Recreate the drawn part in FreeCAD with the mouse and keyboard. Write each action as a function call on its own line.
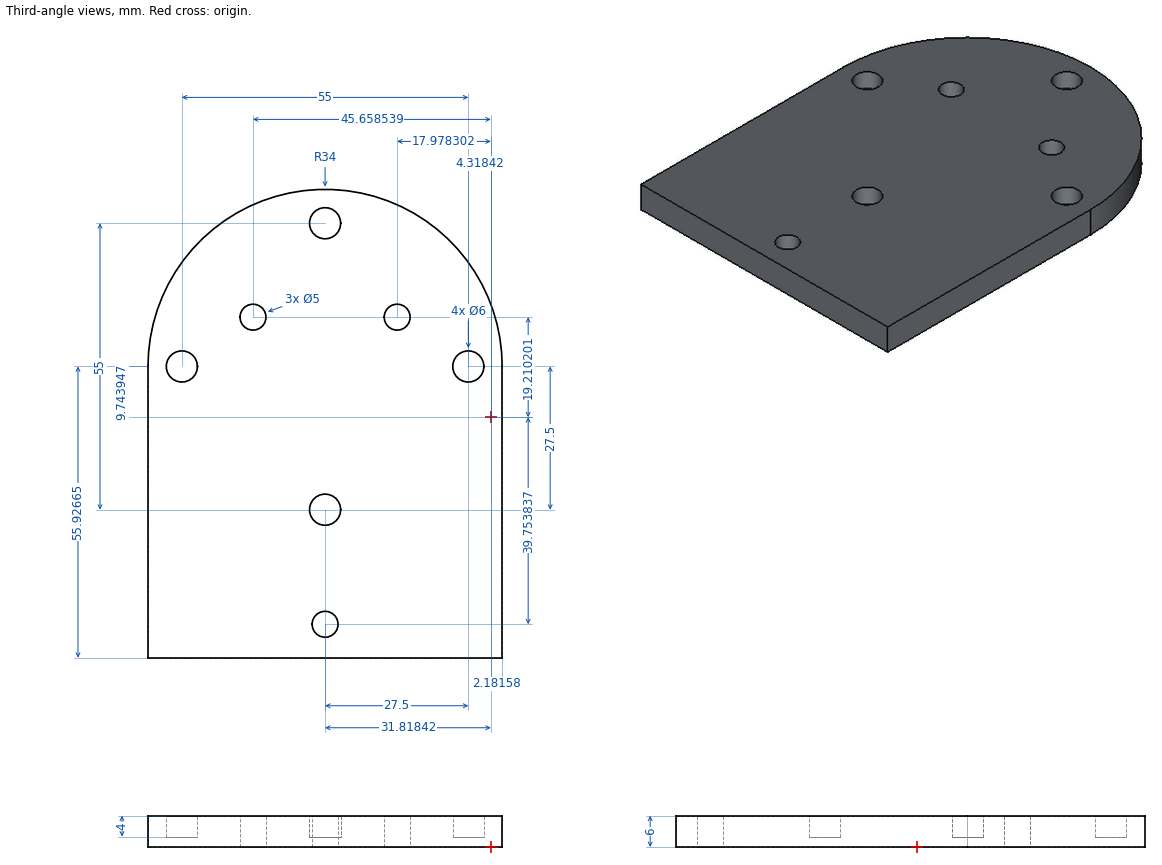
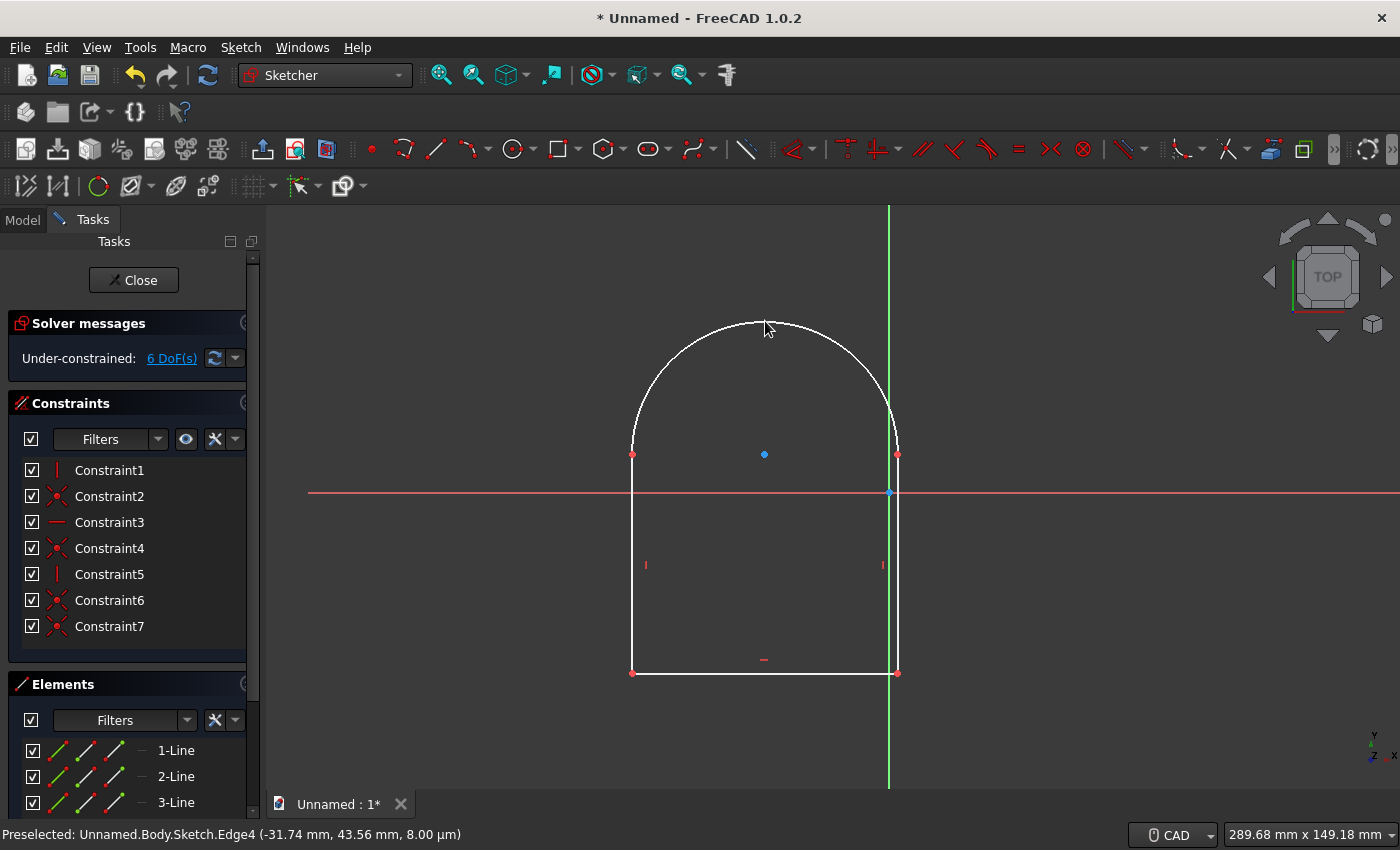
click(632, 521)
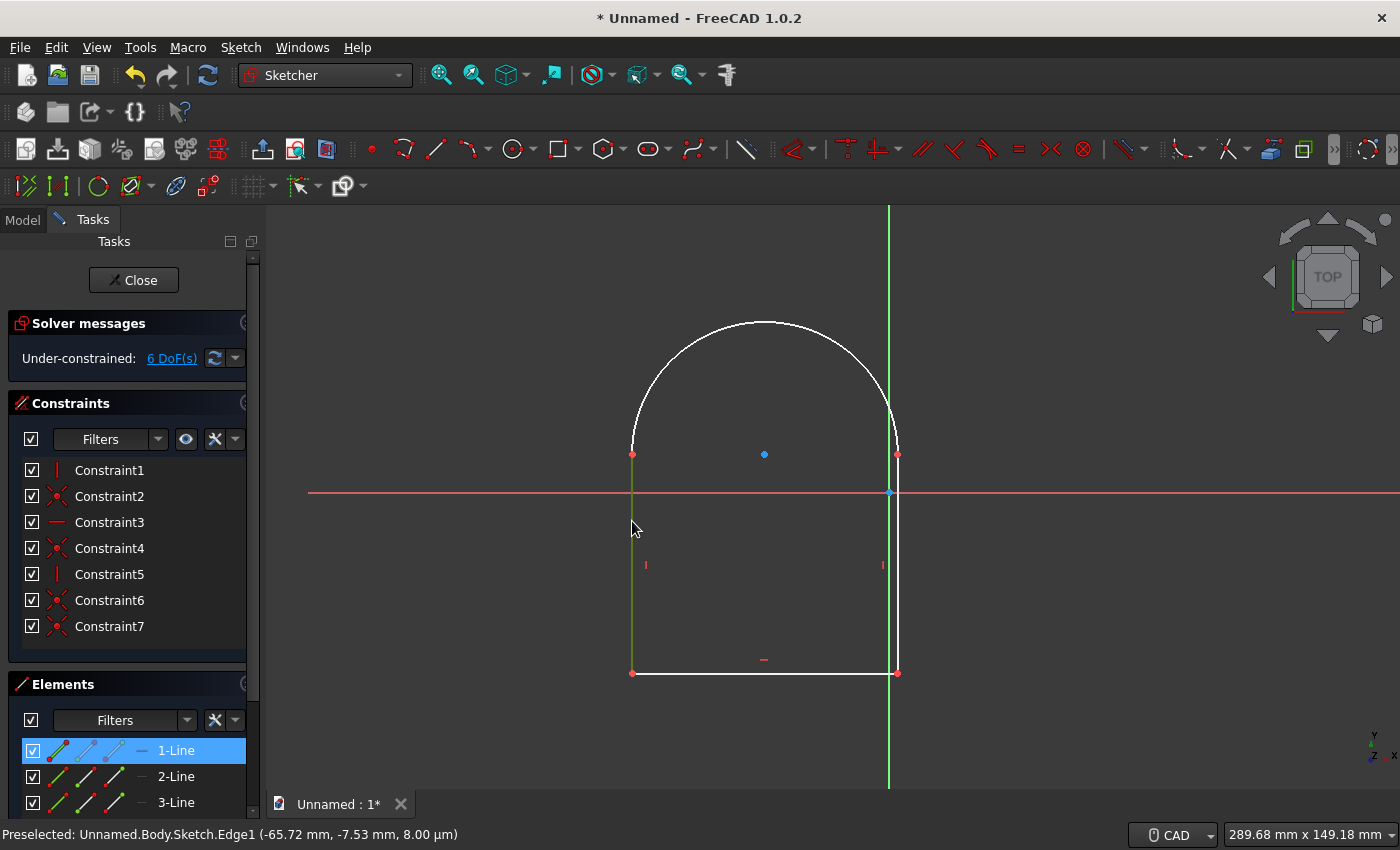
click(843, 347)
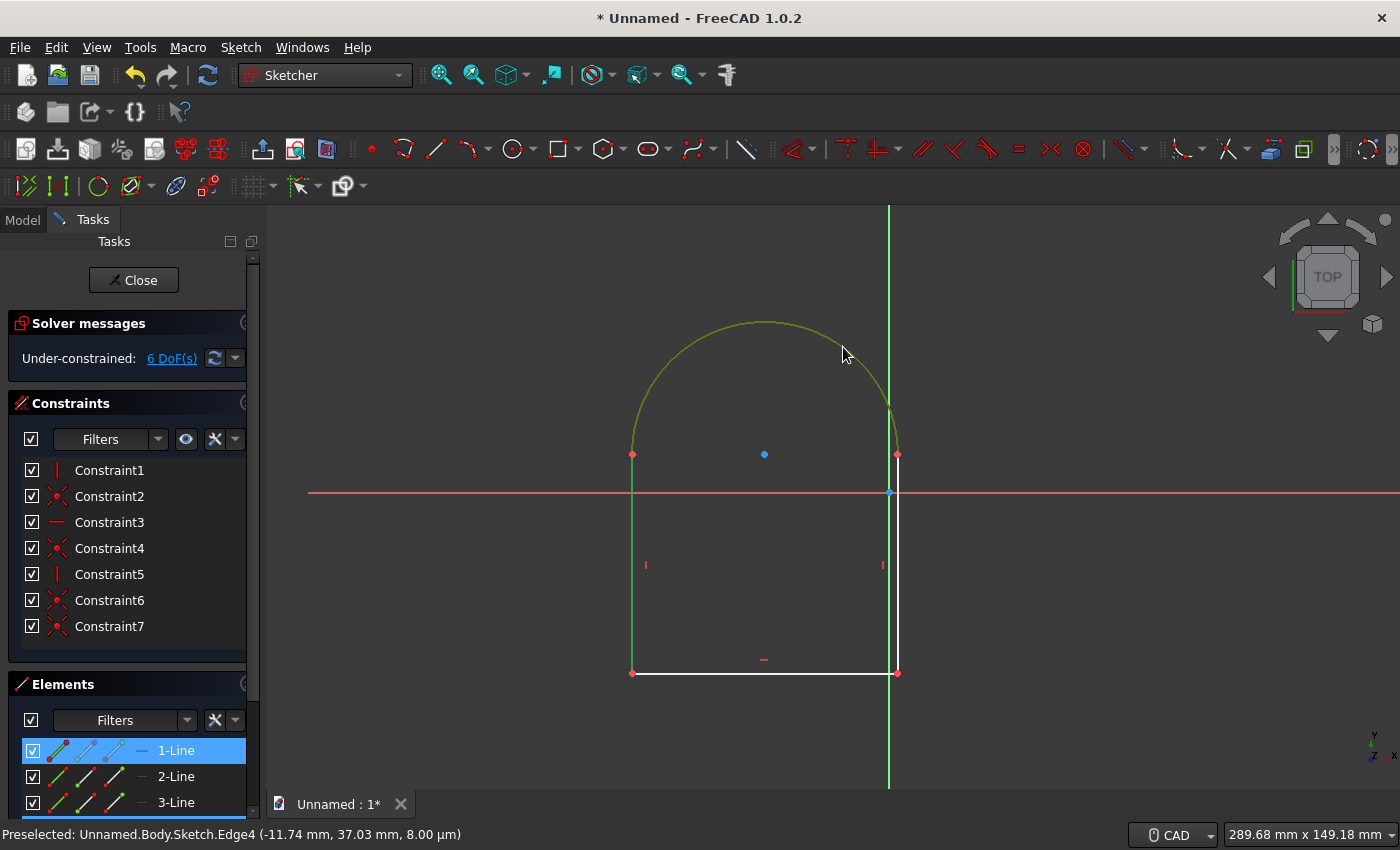
key(t)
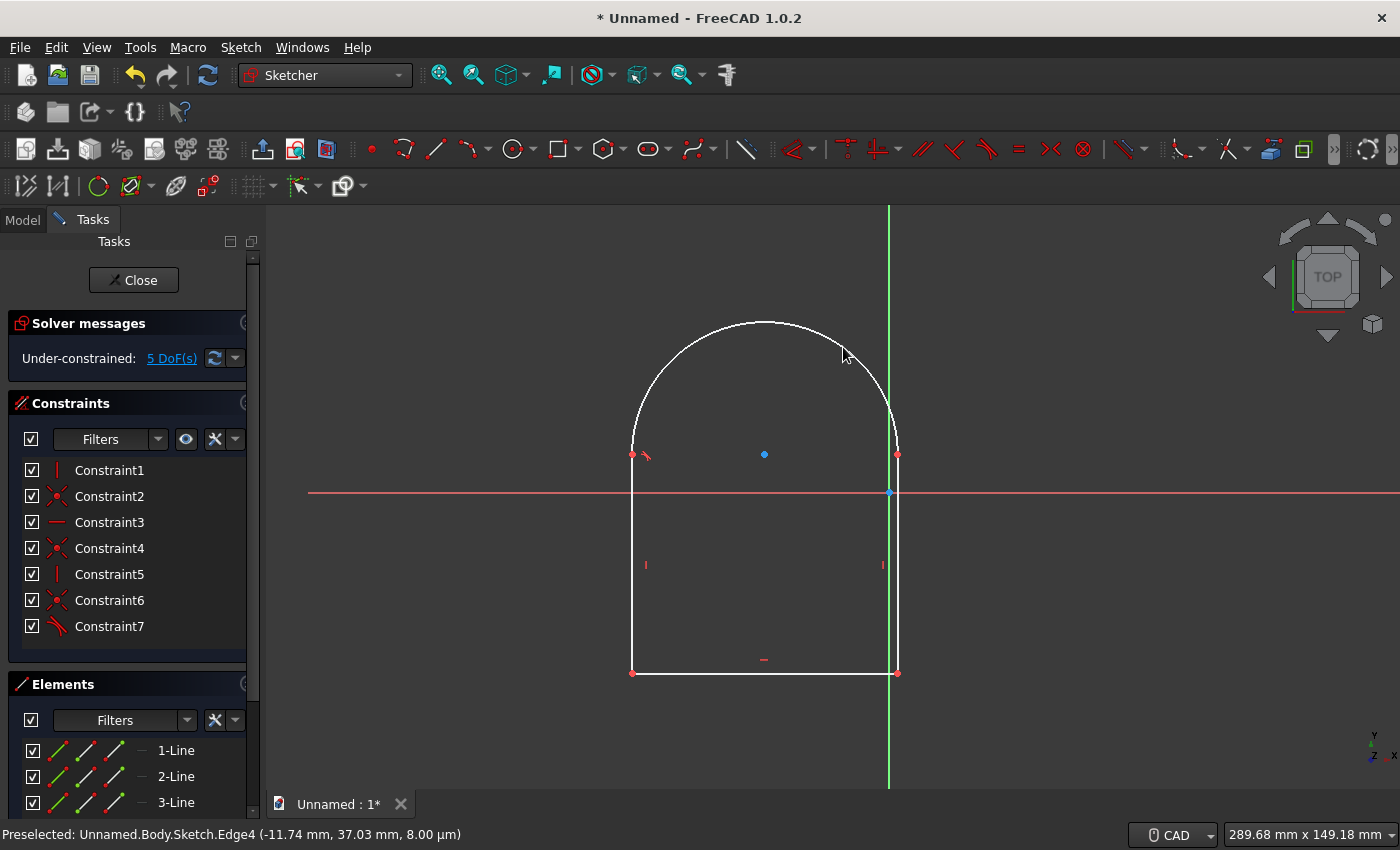
scroll(898, 608, up, 3)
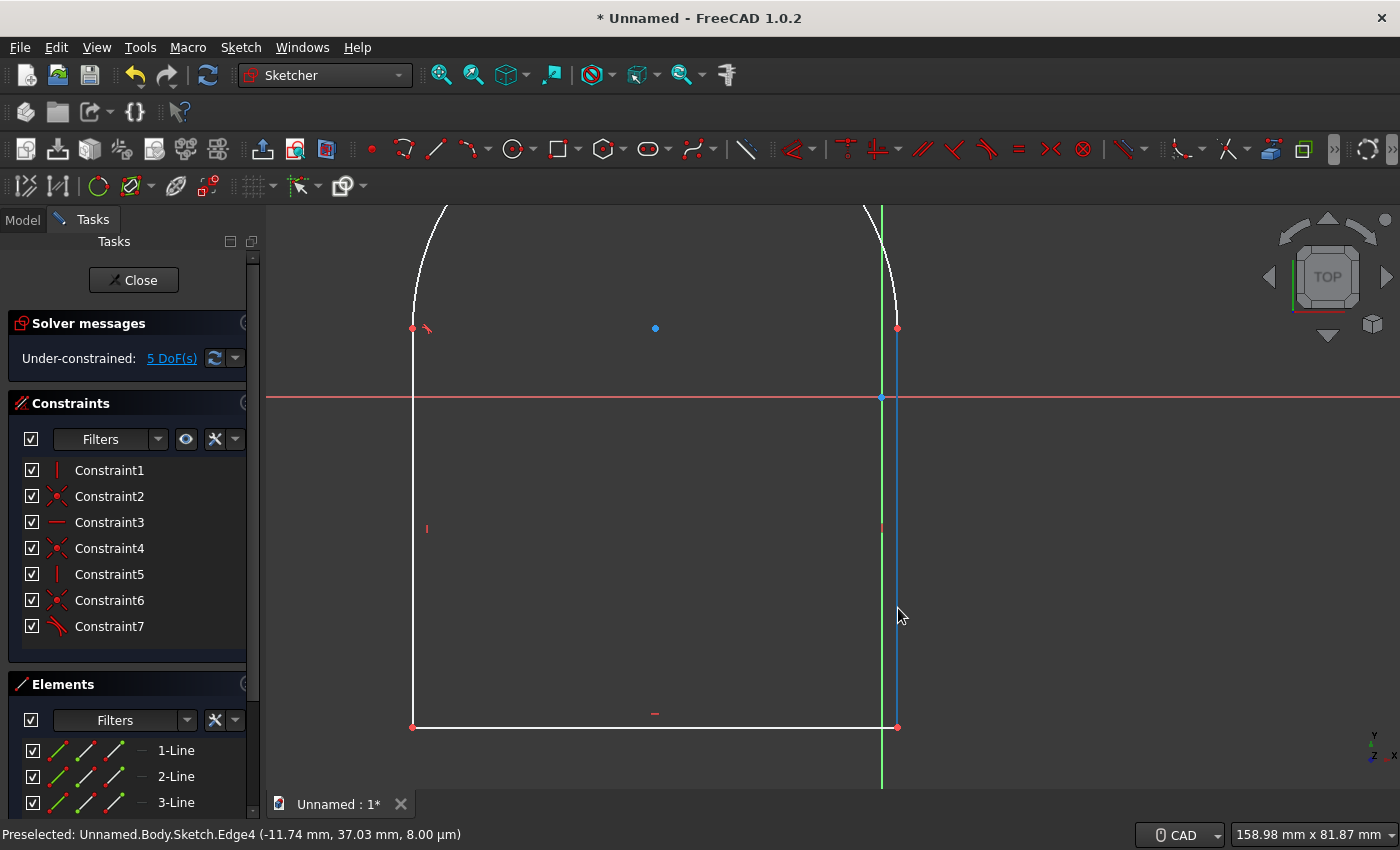
click(897, 608)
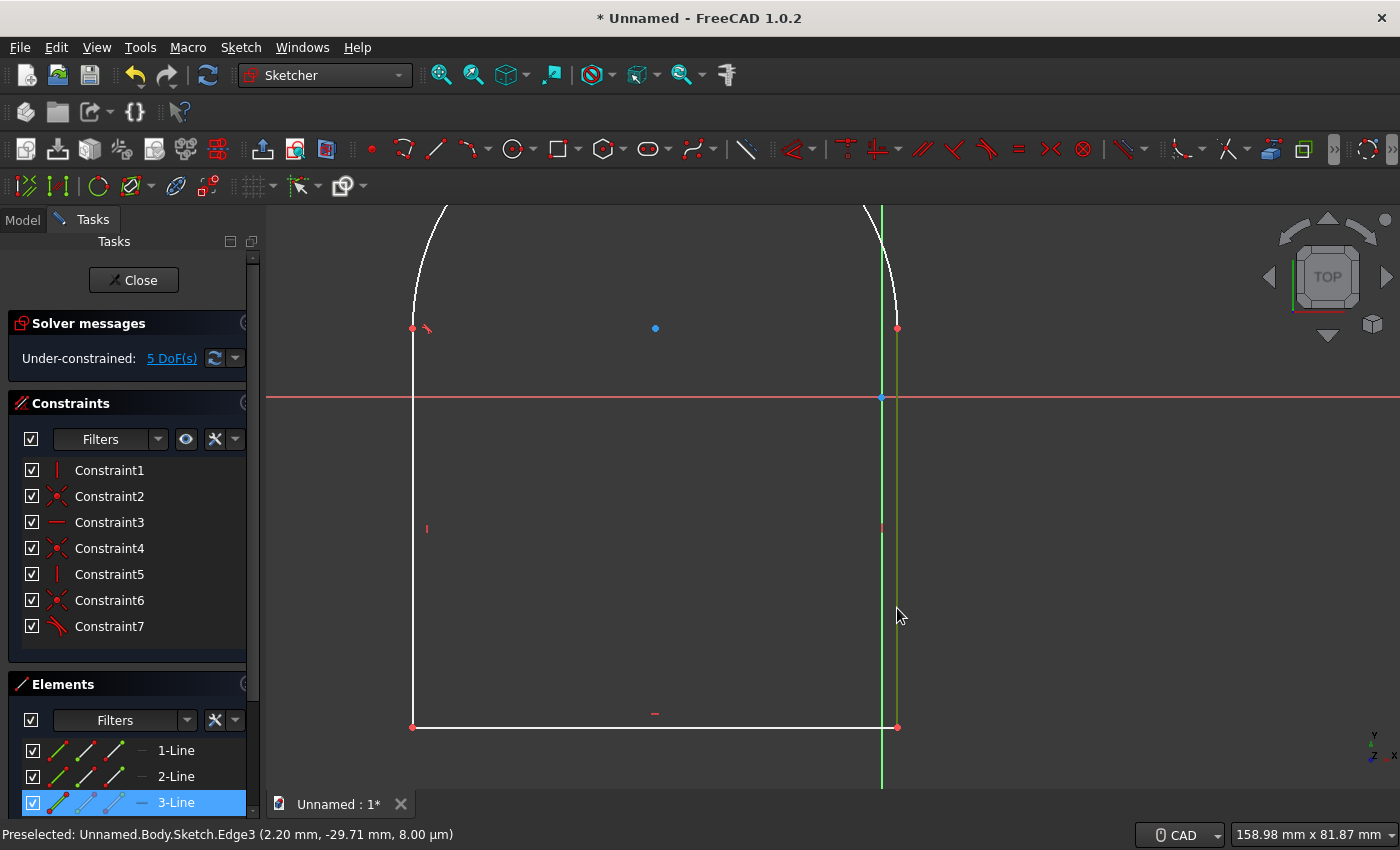
scroll(898, 608, down, 3)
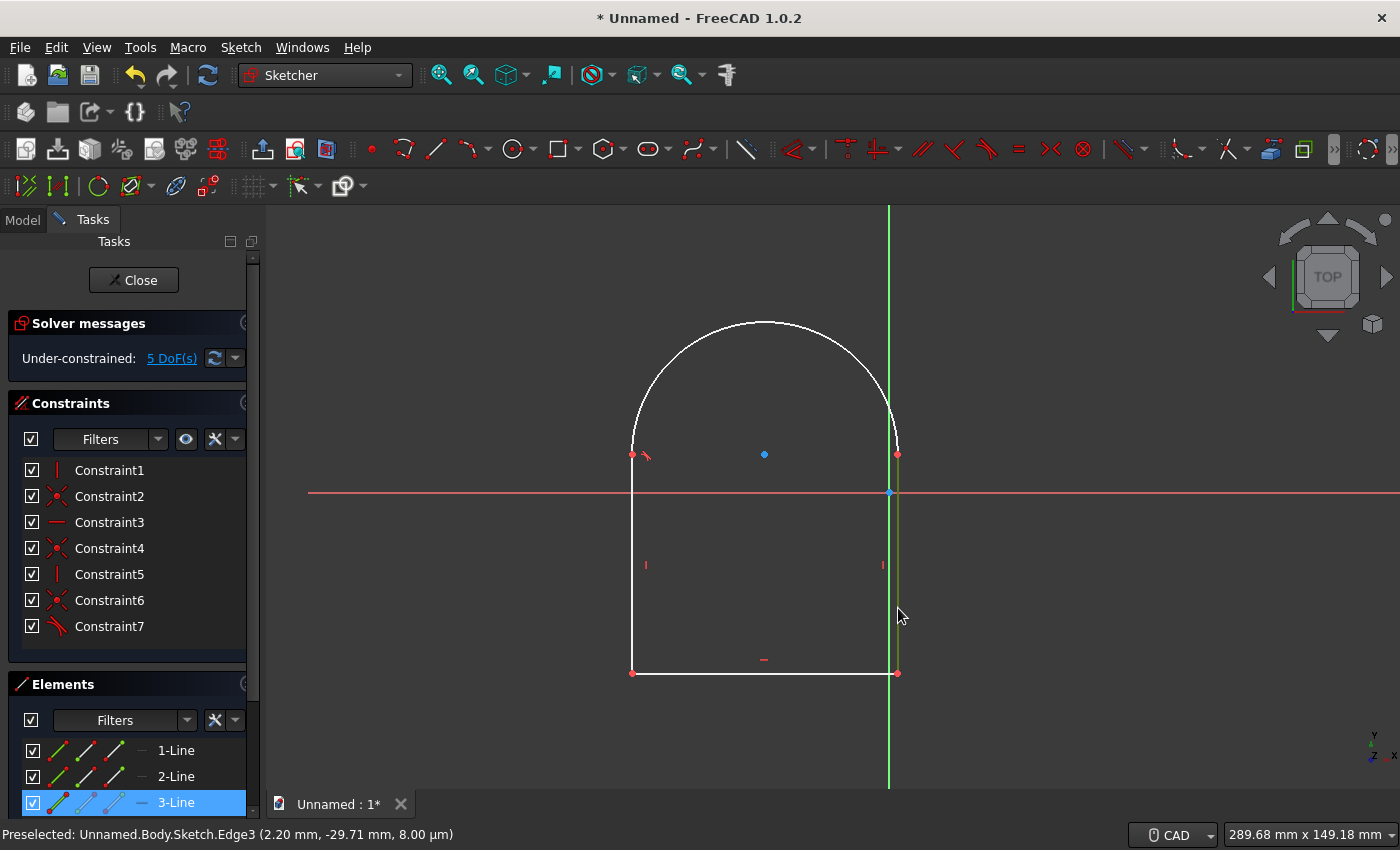
click(843, 347)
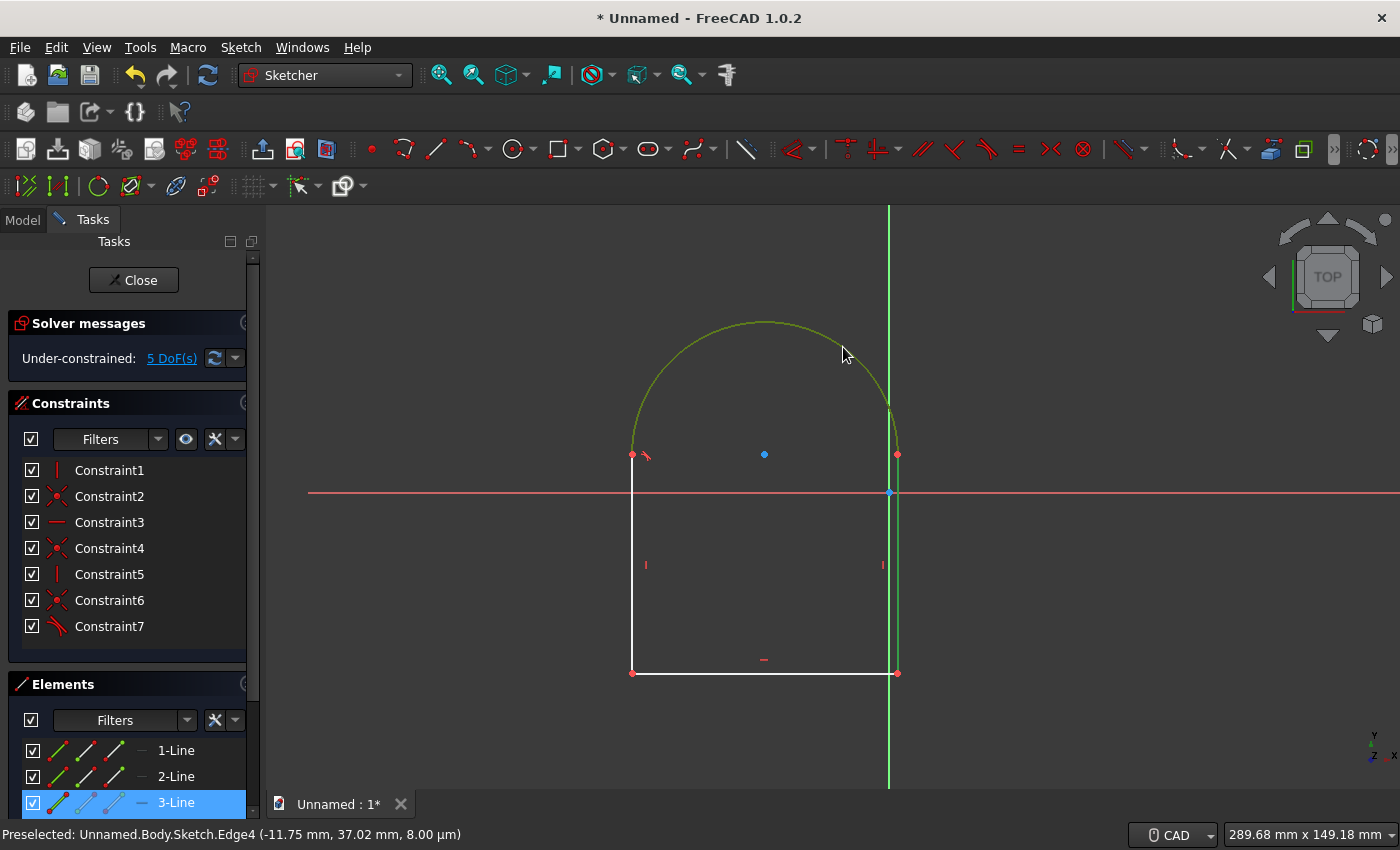
key(t)